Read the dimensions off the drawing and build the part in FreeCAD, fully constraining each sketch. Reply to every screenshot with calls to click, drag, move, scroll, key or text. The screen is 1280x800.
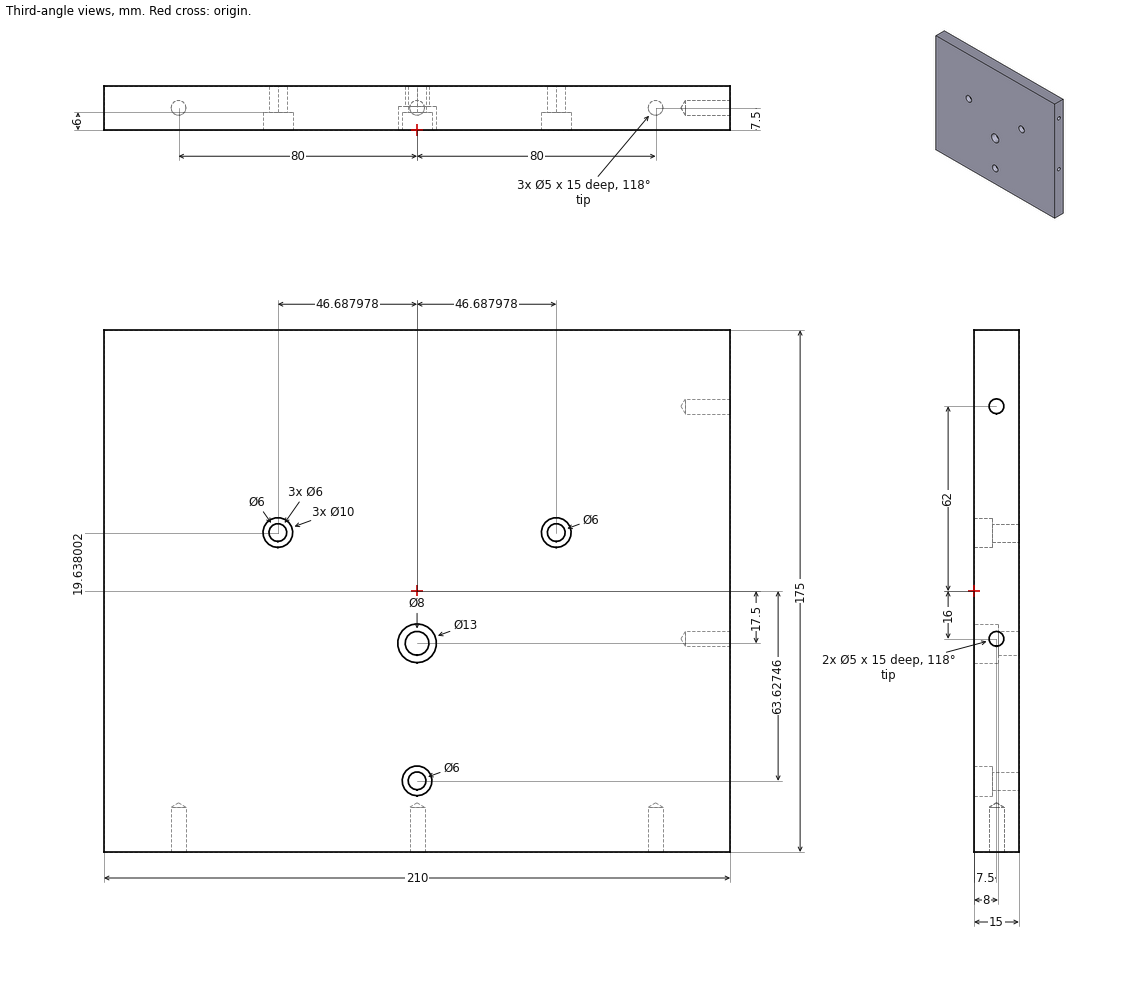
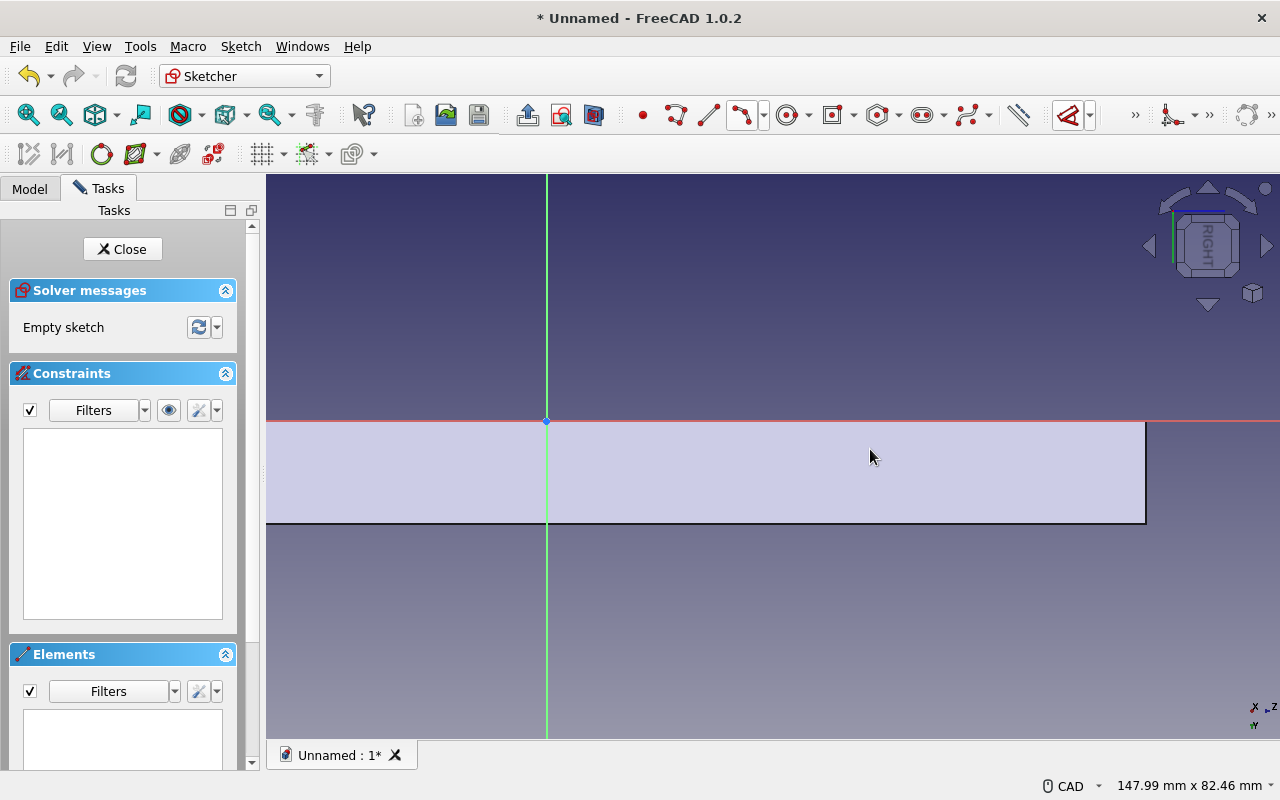
click(786, 116)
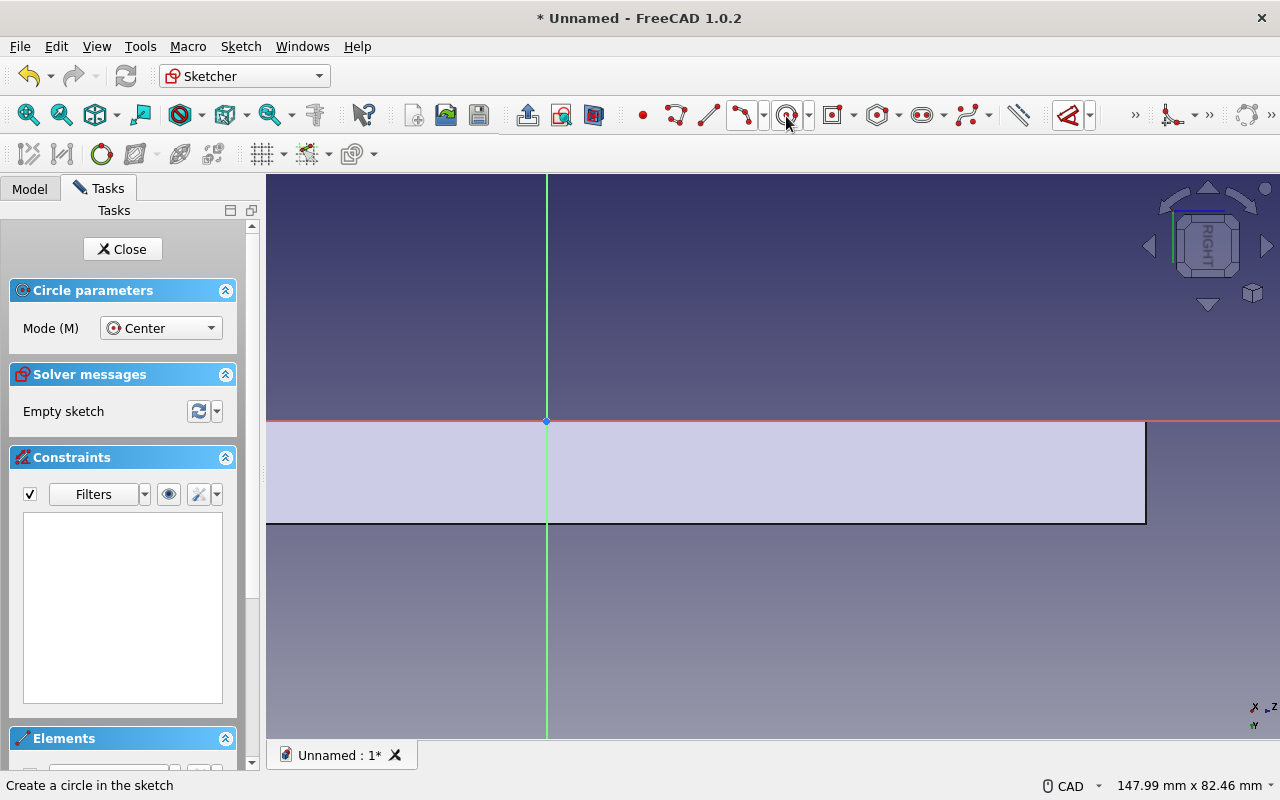
scroll(437, 473, up, 2)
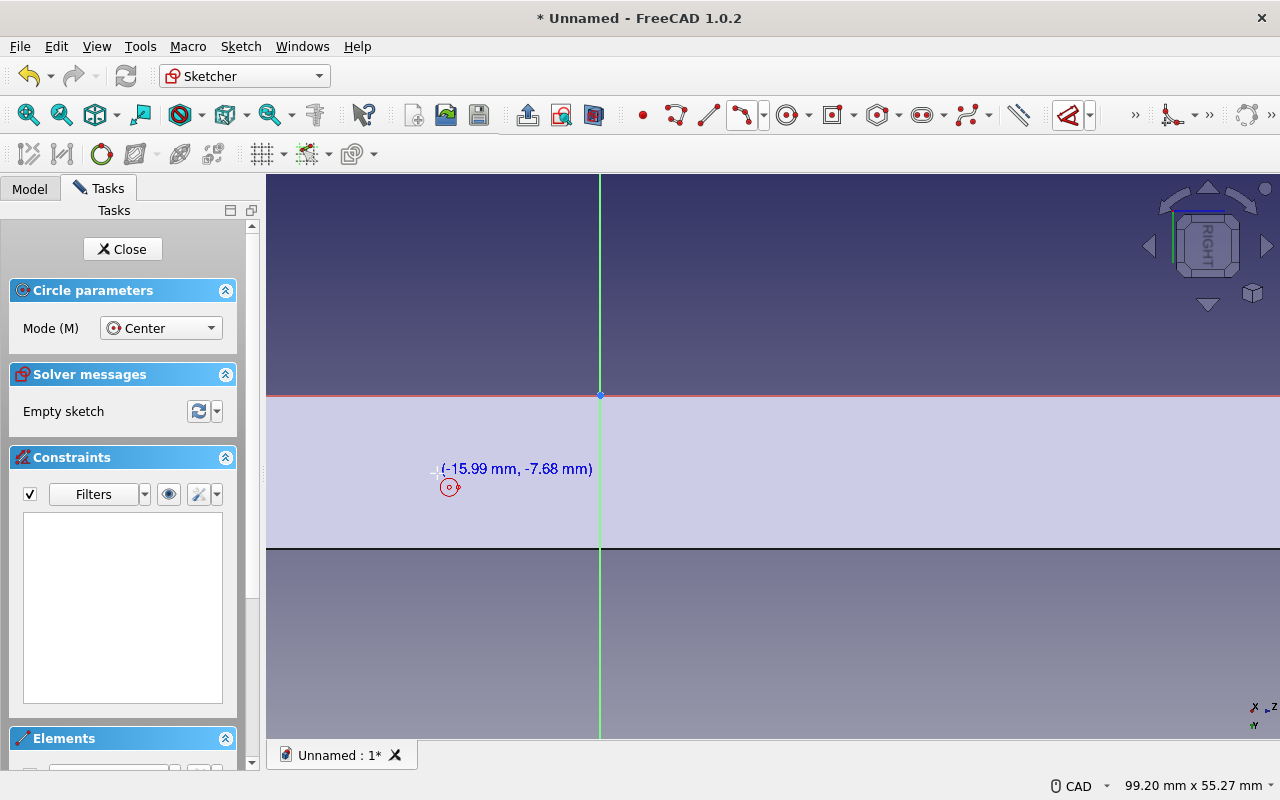
click(437, 472)
click(455, 454)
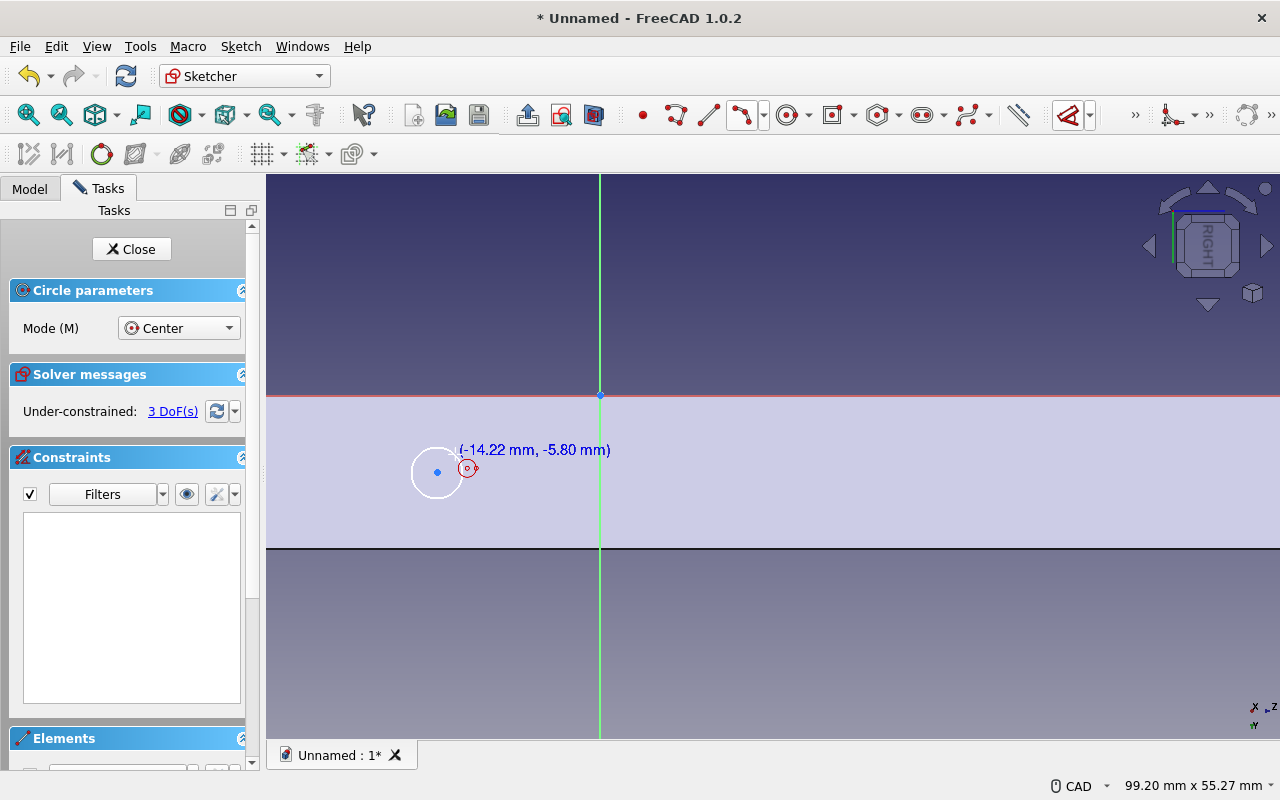
scroll(438, 476, down, 2)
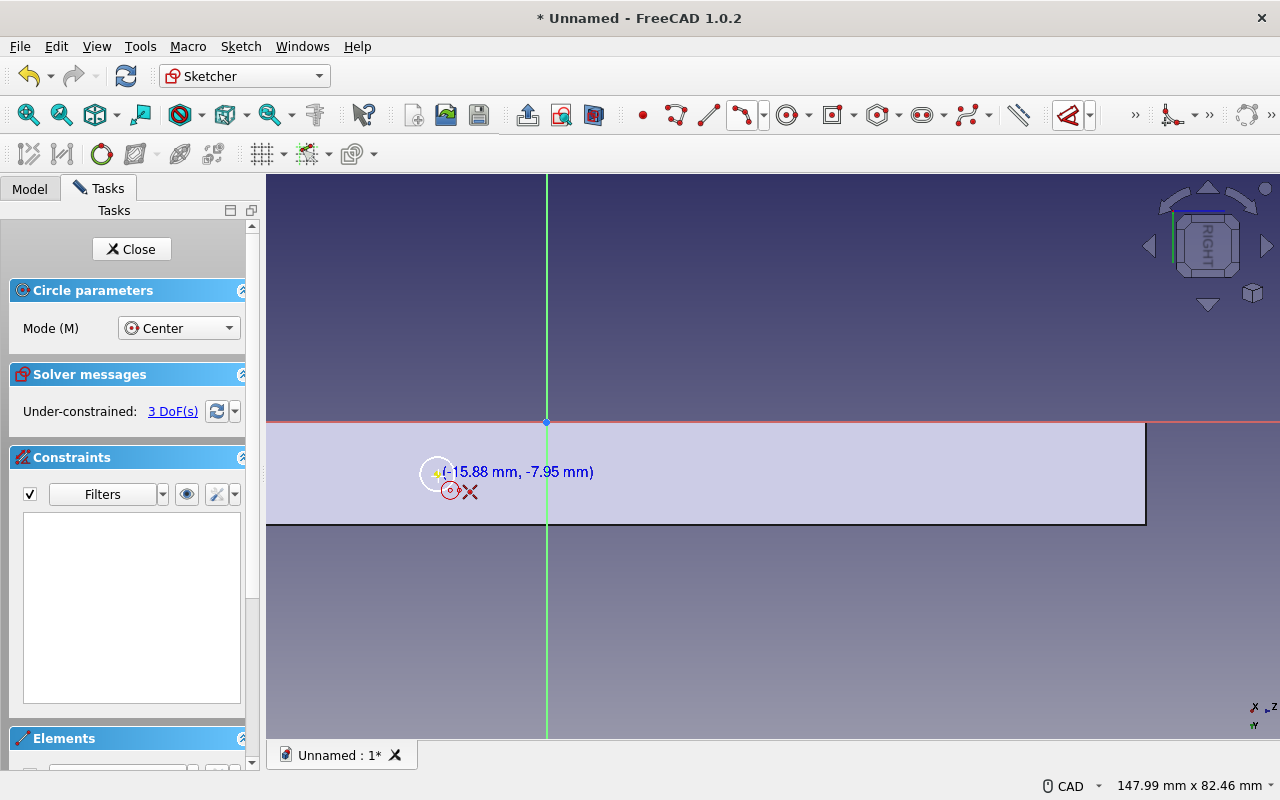
scroll(972, 474, up, 2)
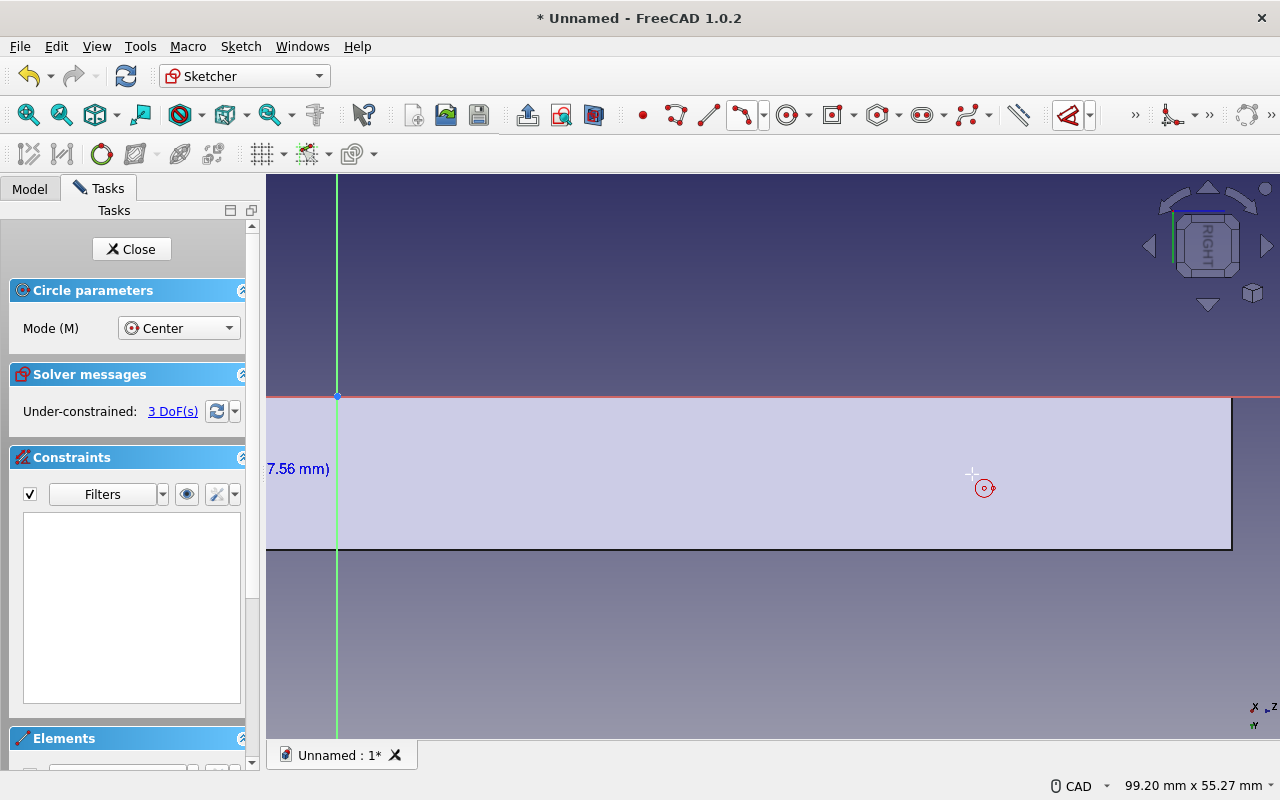
click(971, 473)
click(989, 455)
key(Escape)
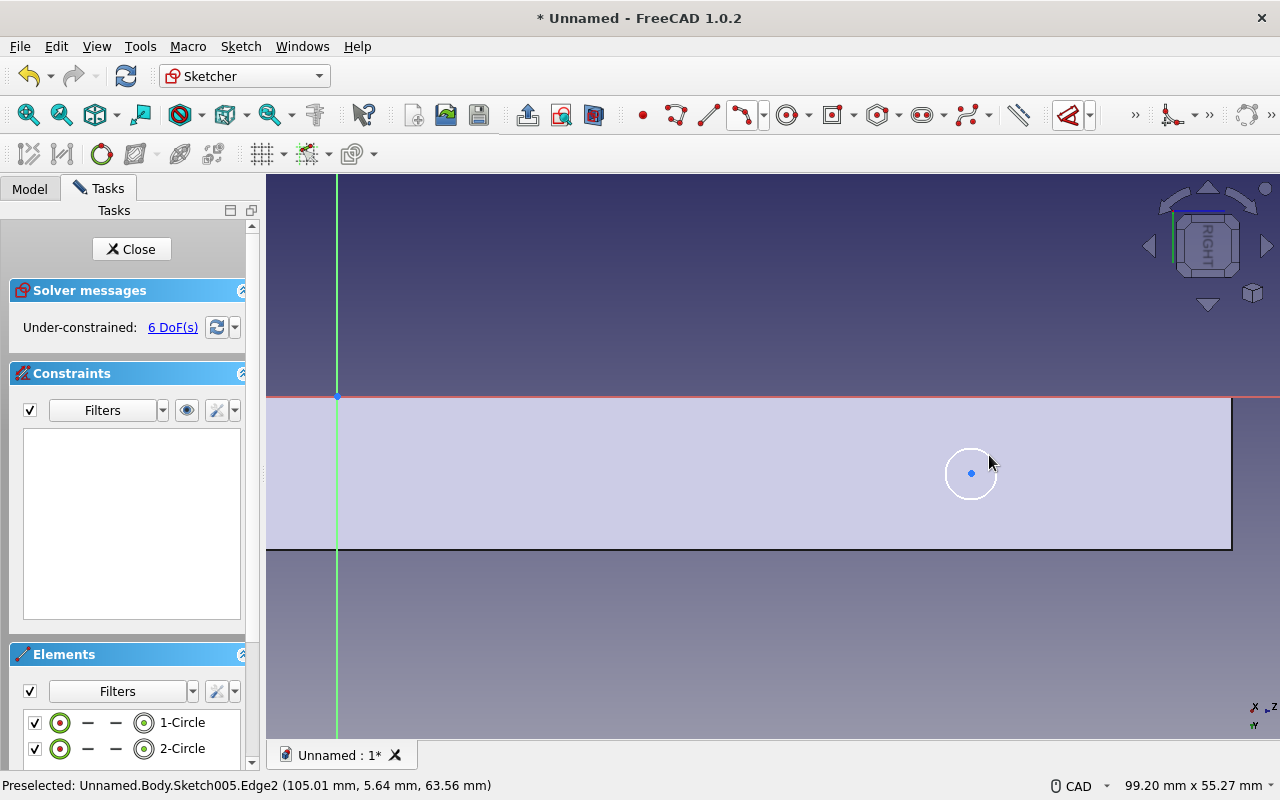
scroll(973, 474, down, 2)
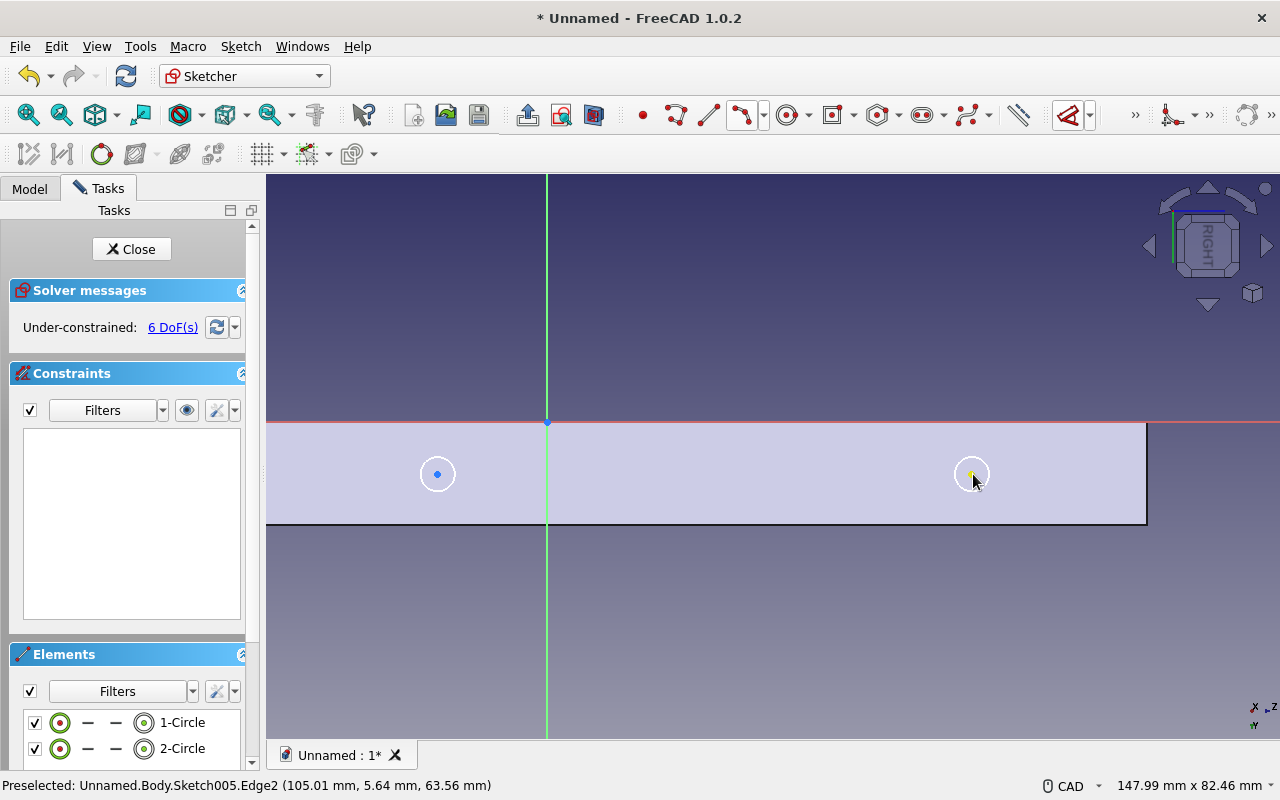
click(450, 462)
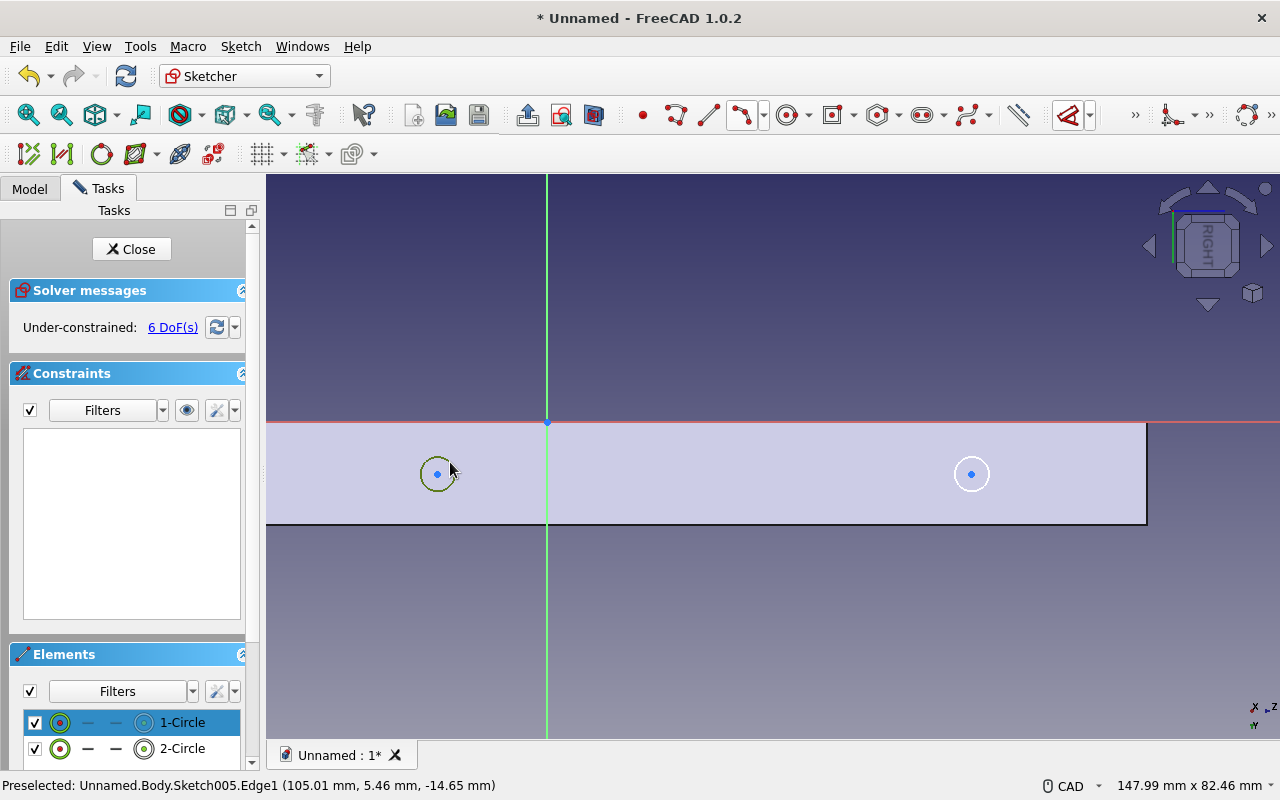
click(984, 462)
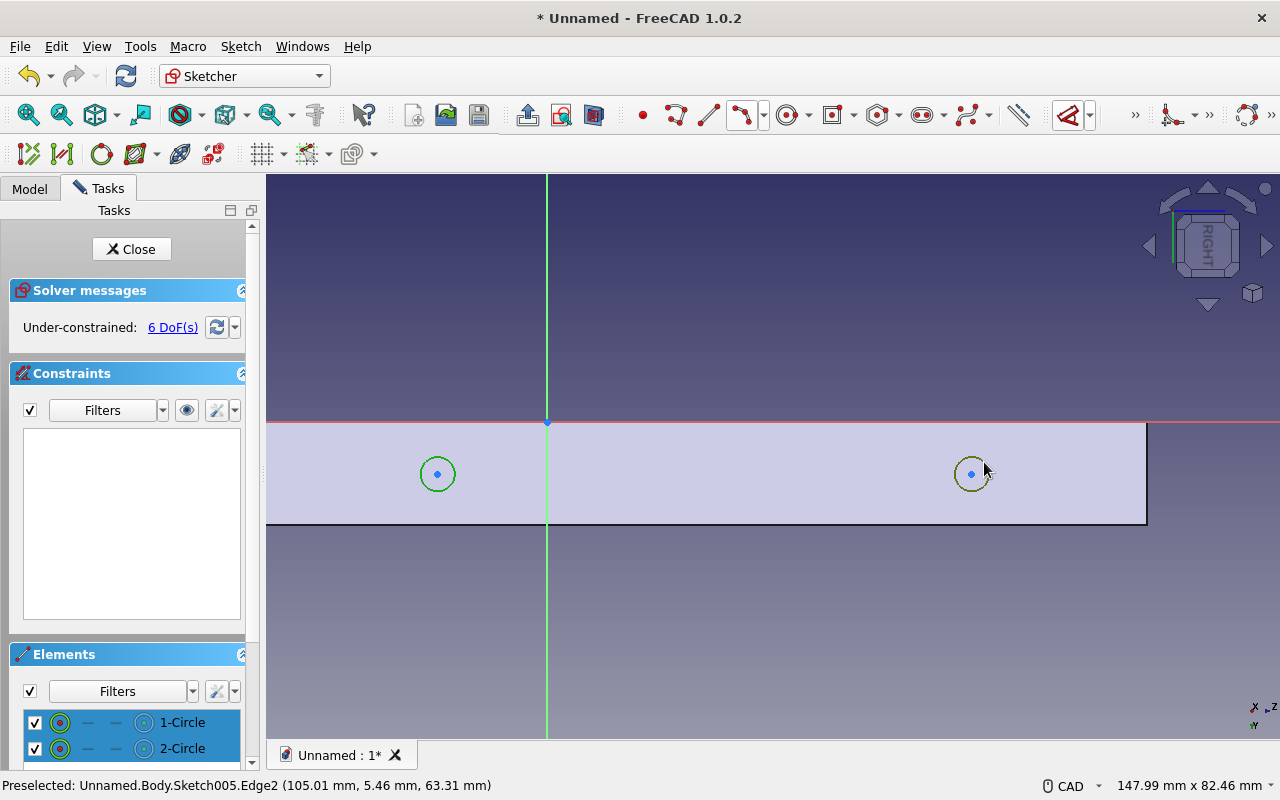
key(e)